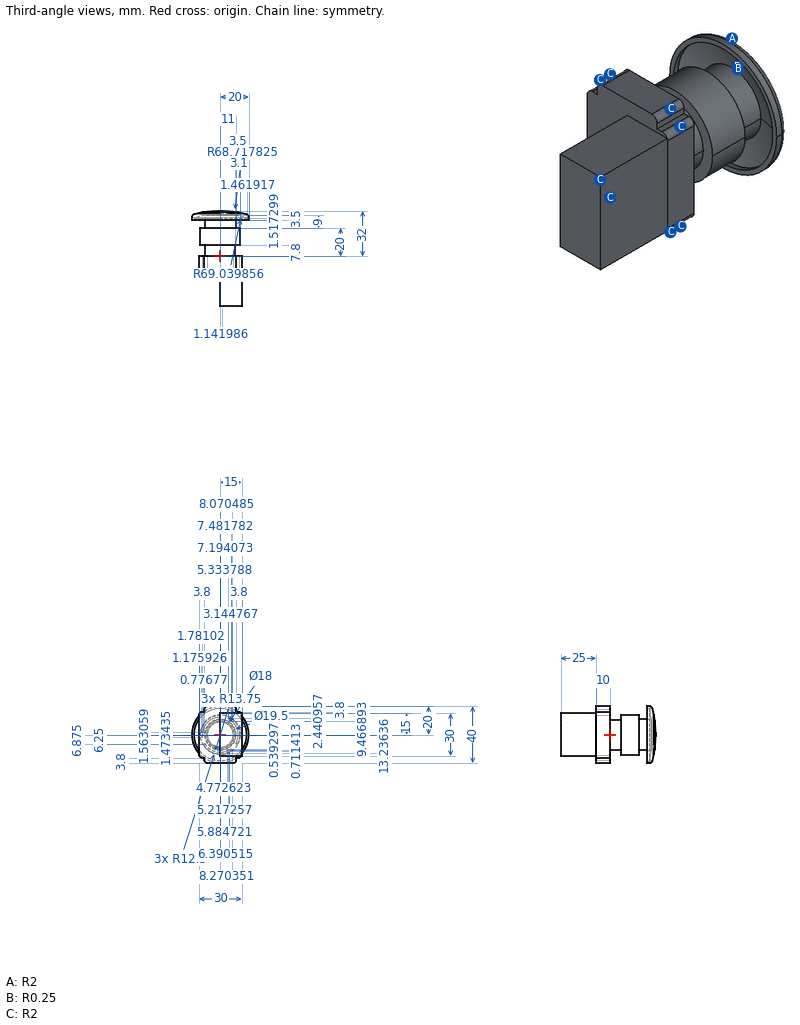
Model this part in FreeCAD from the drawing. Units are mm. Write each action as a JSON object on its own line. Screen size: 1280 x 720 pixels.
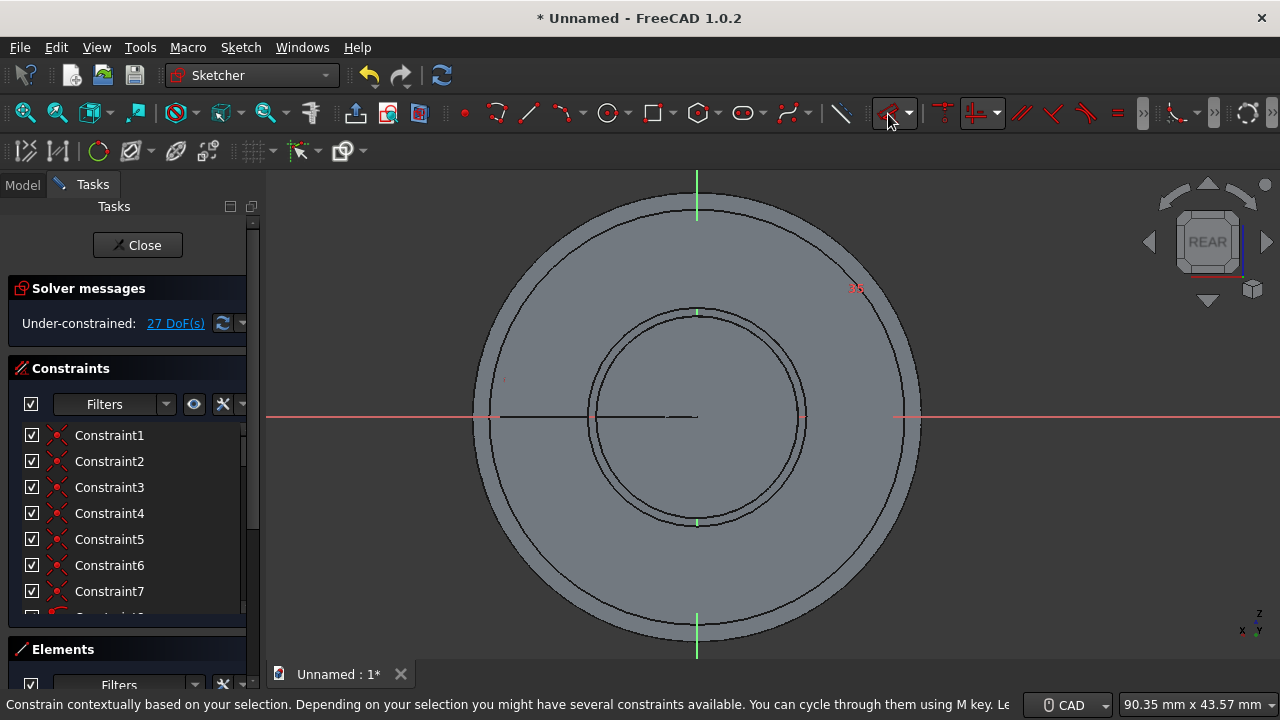
{"action": "left_click", "coordinate": [698, 557]}
{"action": "left_click", "coordinate": [780, 567]}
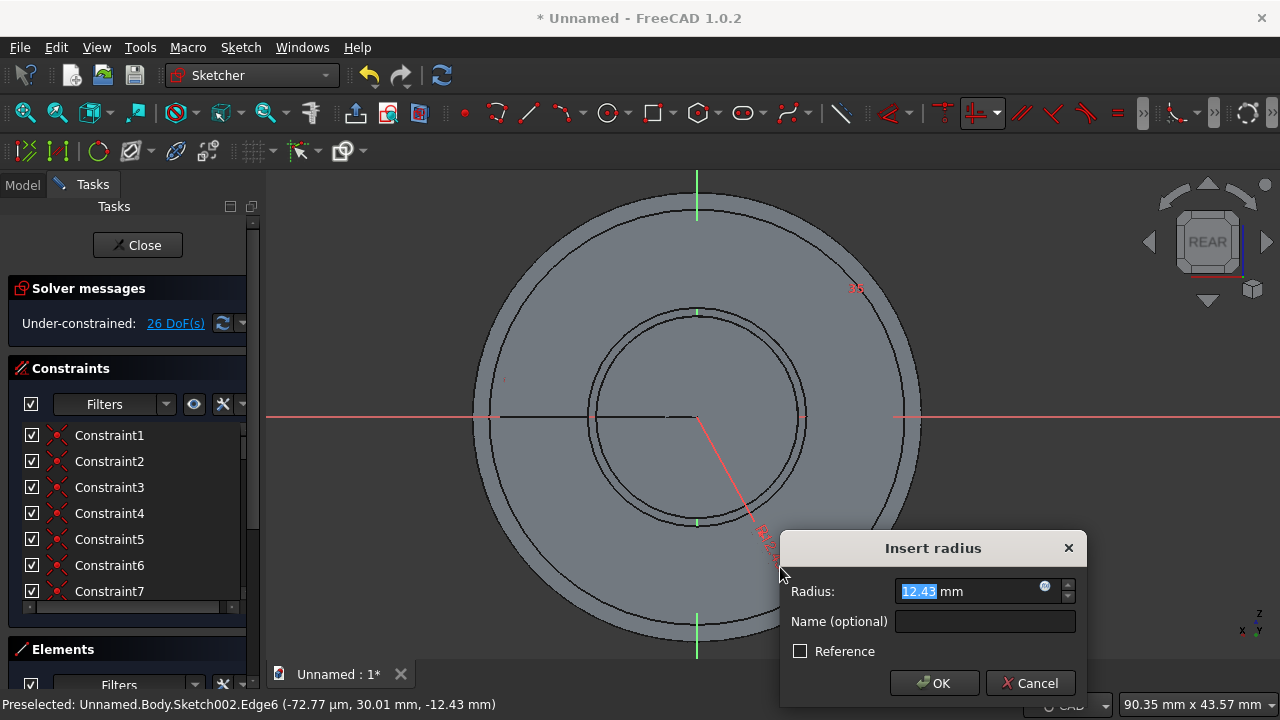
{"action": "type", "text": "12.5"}
{"action": "key", "text": "Return"}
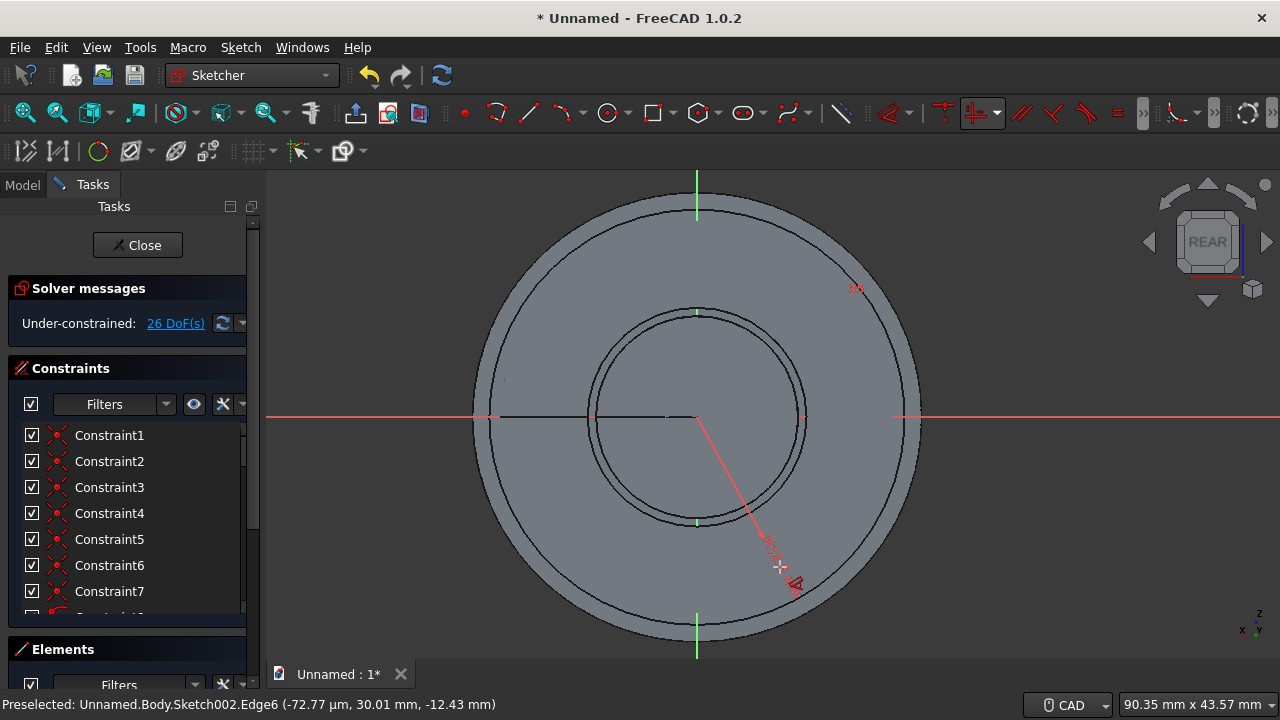
{"action": "left_click", "coordinate": [697, 571]}
{"action": "left_click", "coordinate": [608, 580]}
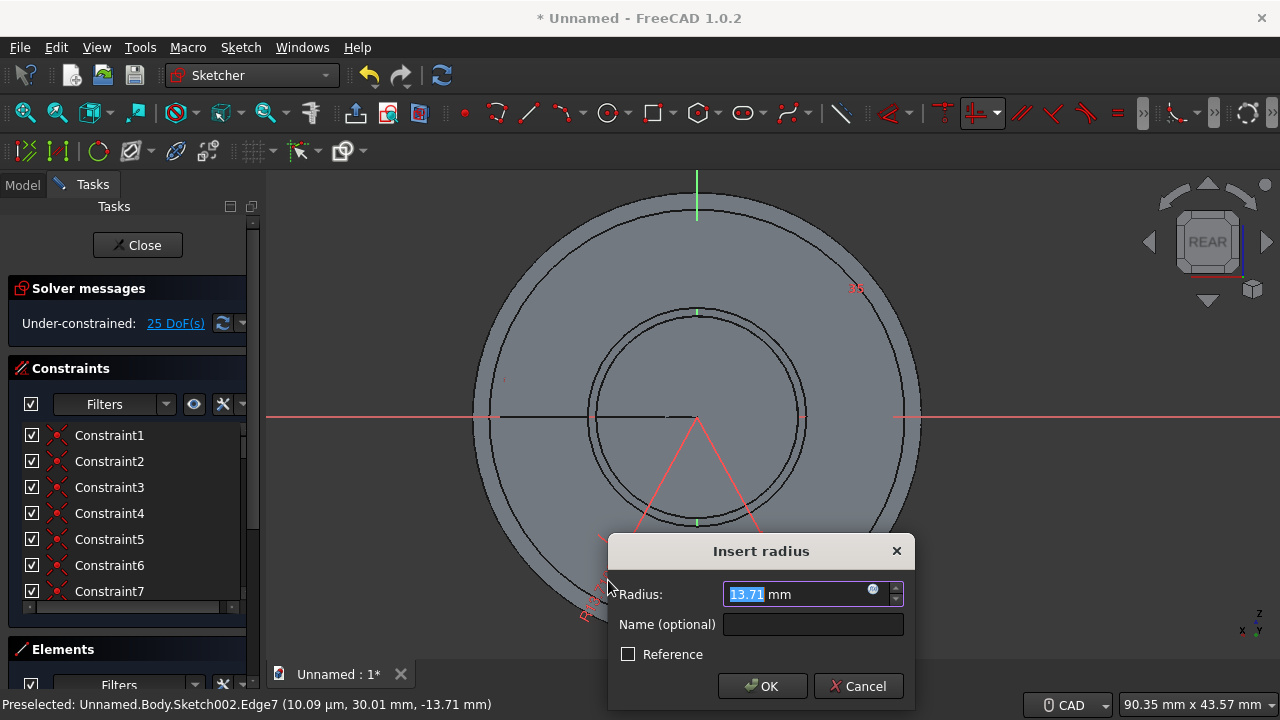
{"action": "type", "text": "13.75"}
{"action": "key", "text": "Return"}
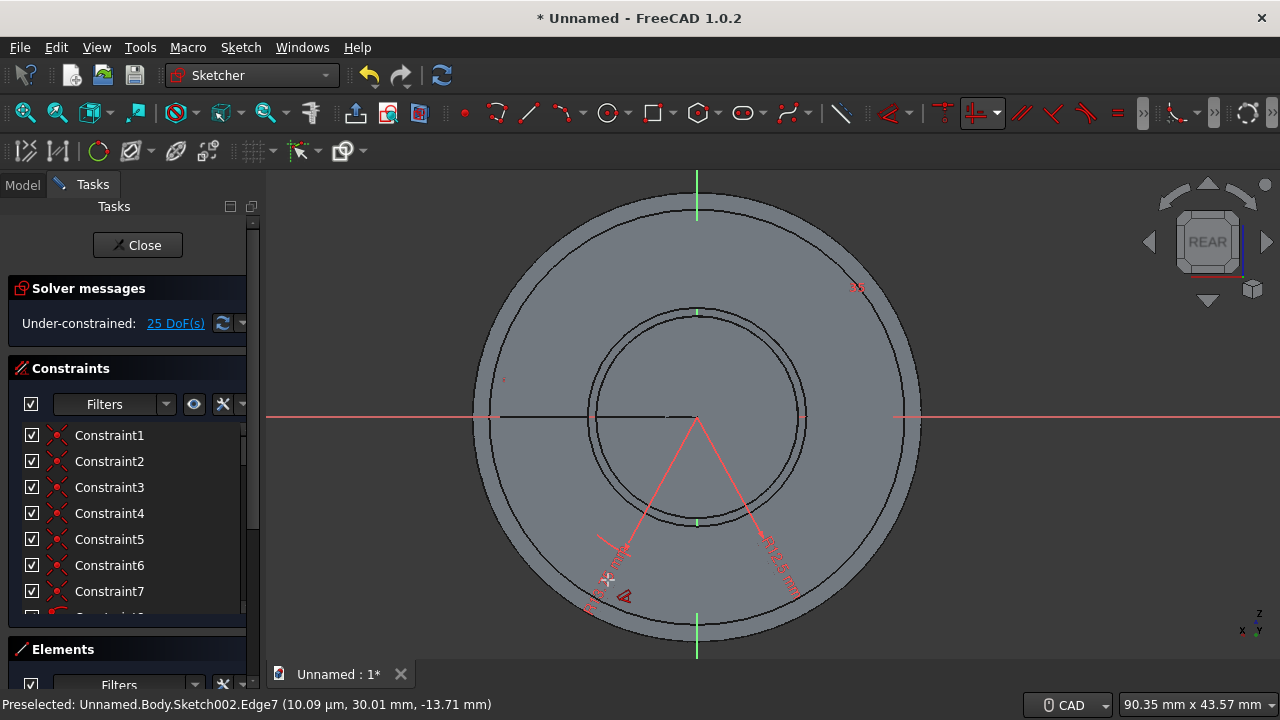
{"action": "left_click", "coordinate": [818, 489]}
{"action": "left_click", "coordinate": [852, 453]}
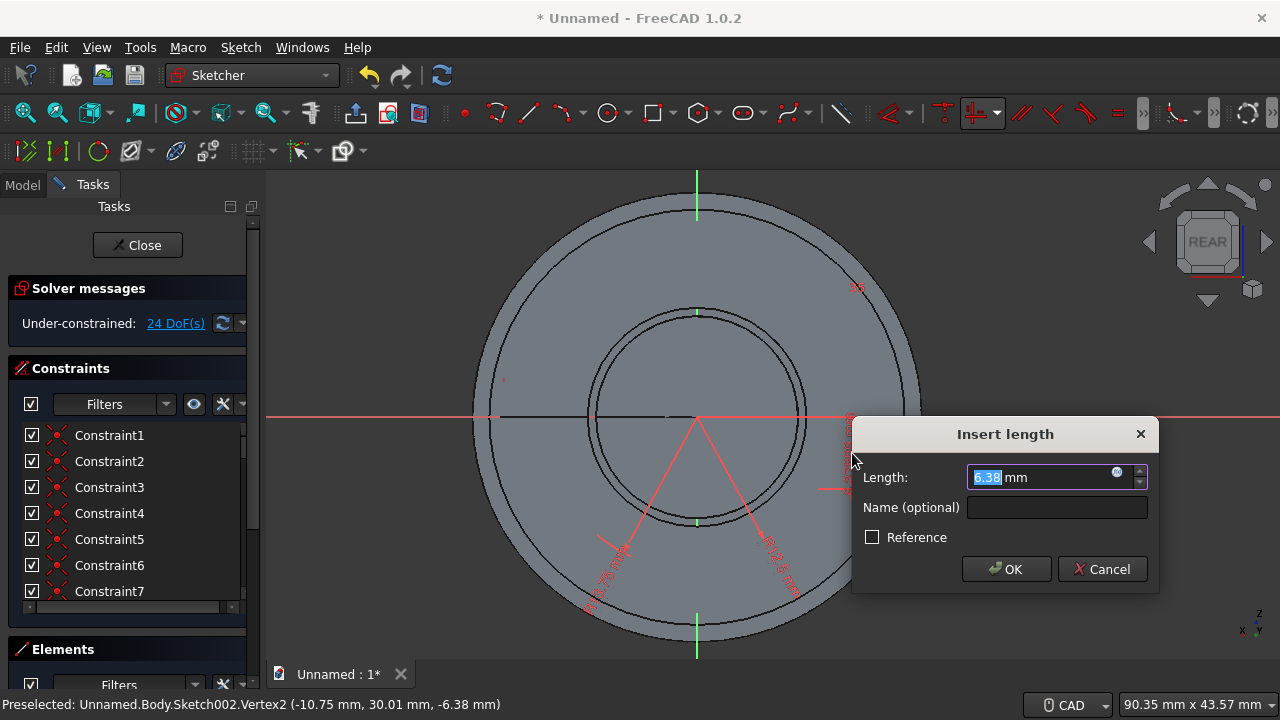
{"action": "type", "text": "6.25"}
{"action": "key", "text": "Return"}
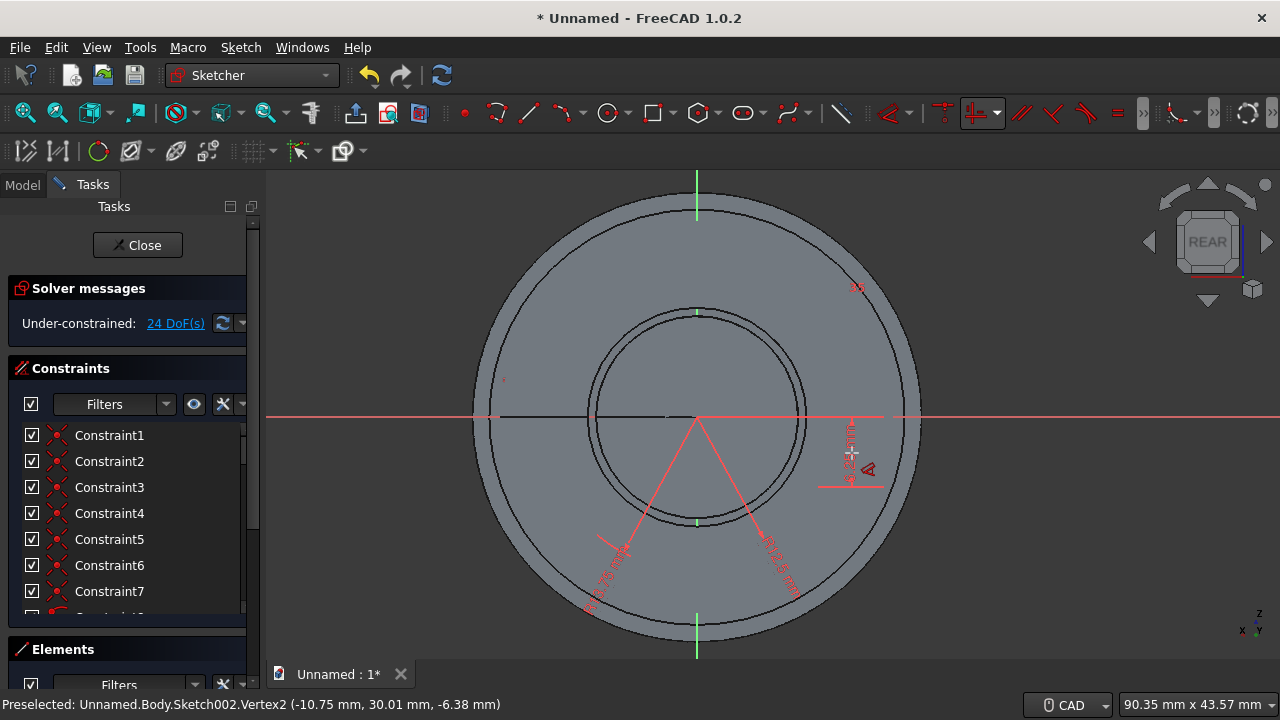
{"action": "left_click", "coordinate": [576, 488]}
{"action": "left_click", "coordinate": [731, 453]}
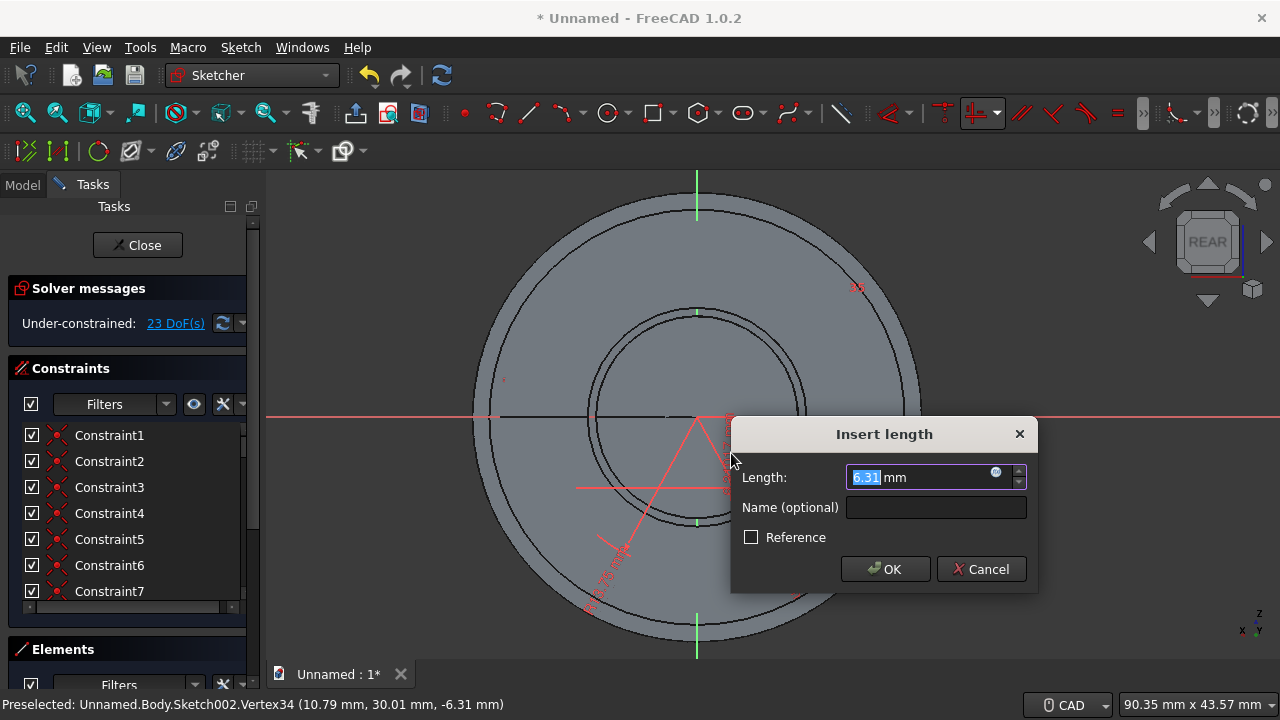
{"action": "type", "text": "6.25"}
{"action": "key", "text": "Return"}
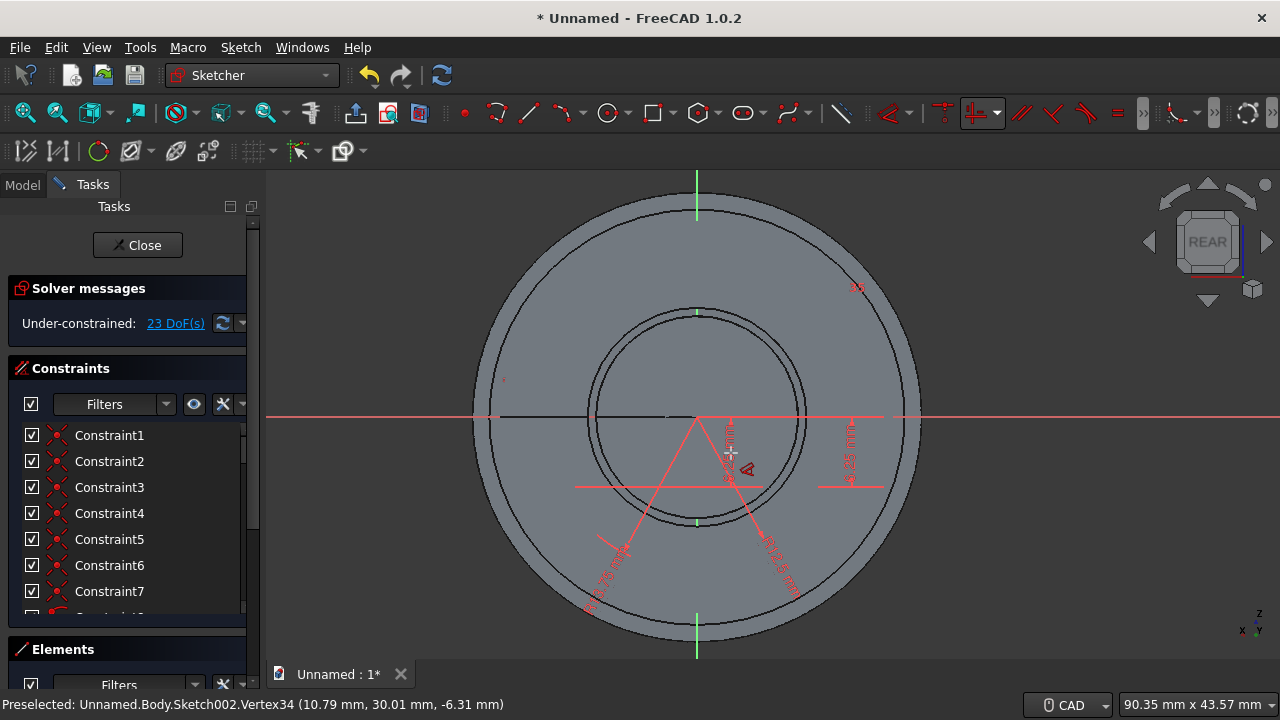
{"action": "left_click", "coordinate": [830, 496]}
{"action": "left_click", "coordinate": [864, 475]}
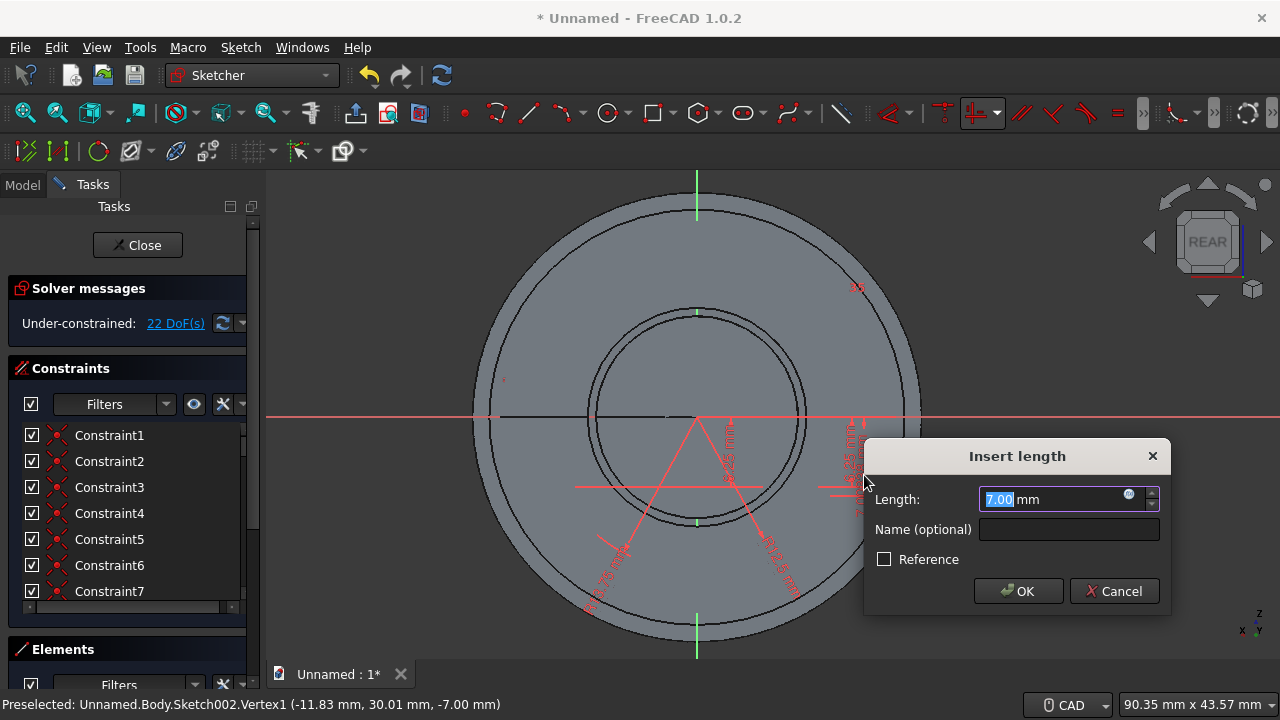
{"action": "type", "text": "6.875"}
{"action": "key", "text": "Return"}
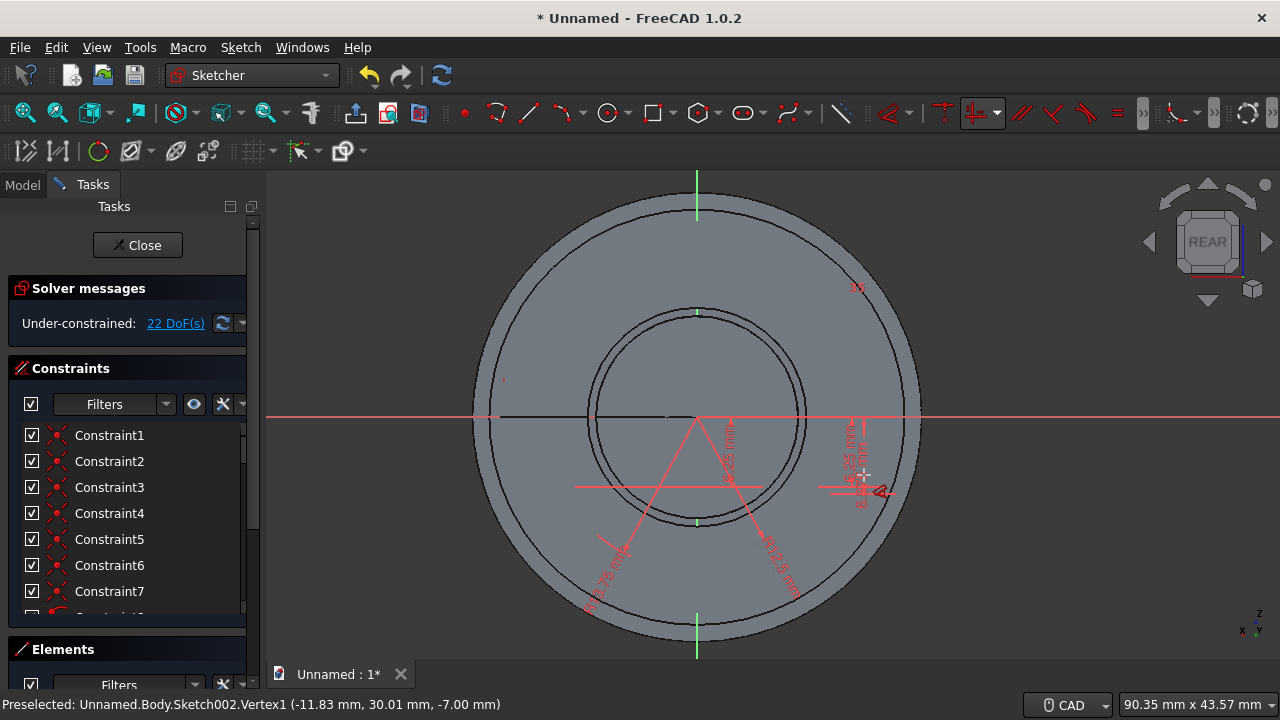
{"action": "left_click", "coordinate": [564, 495]}
{"action": "left_click", "coordinate": [530, 456]}